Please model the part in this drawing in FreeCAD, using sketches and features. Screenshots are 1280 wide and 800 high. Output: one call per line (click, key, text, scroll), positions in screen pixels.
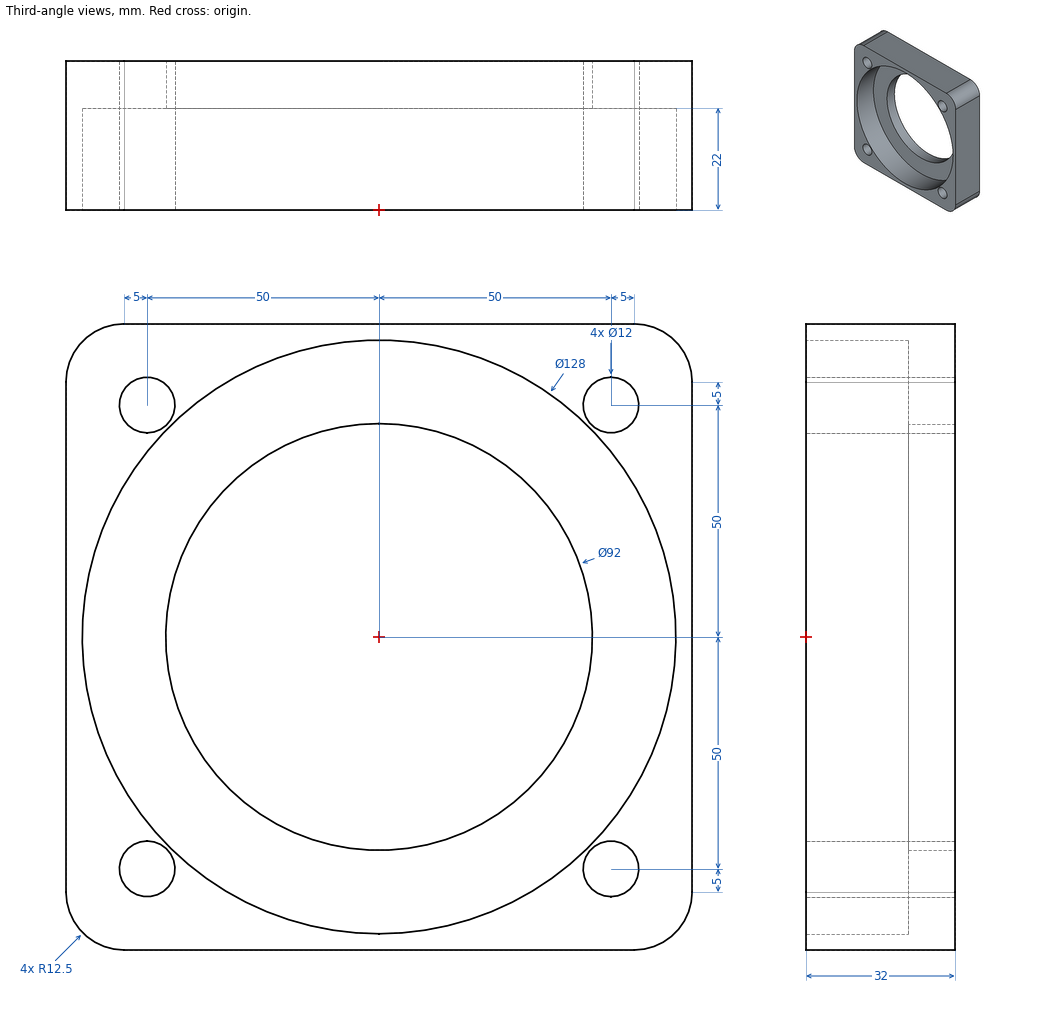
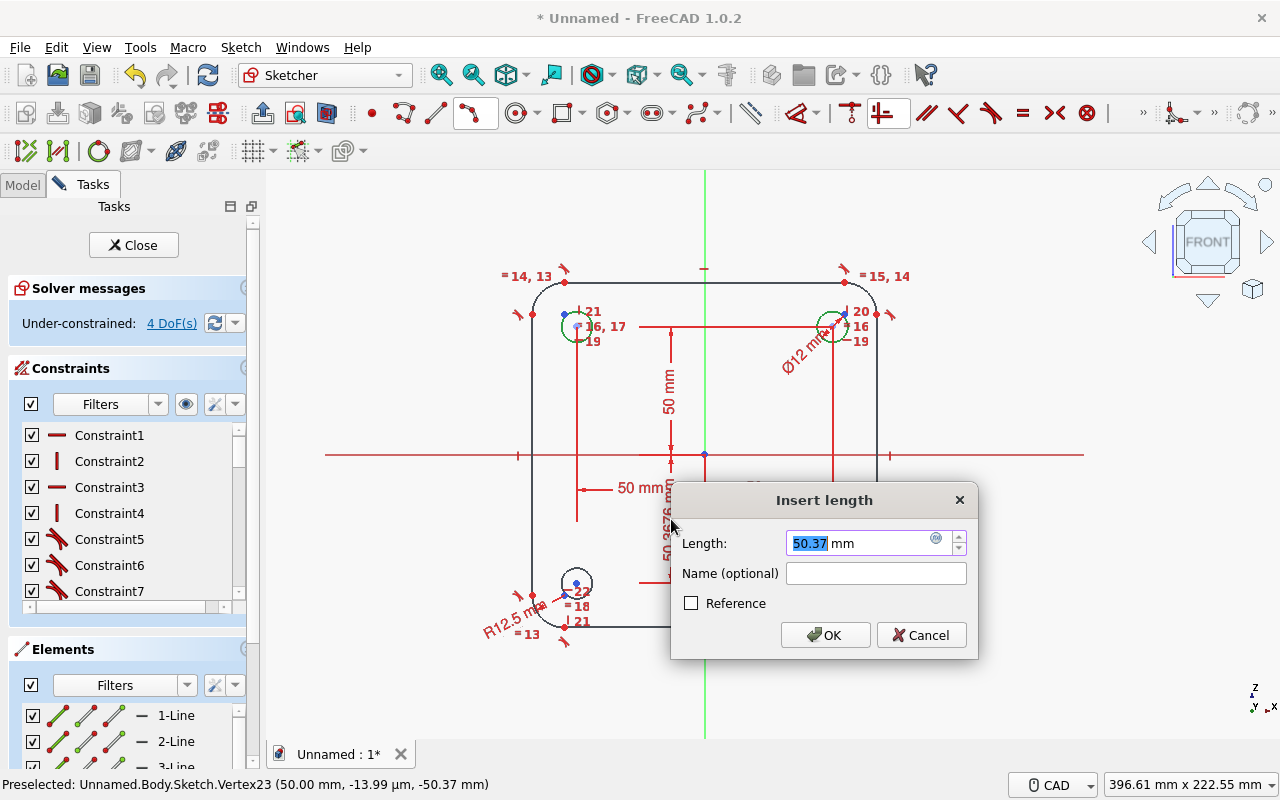
text(50)
key(Return)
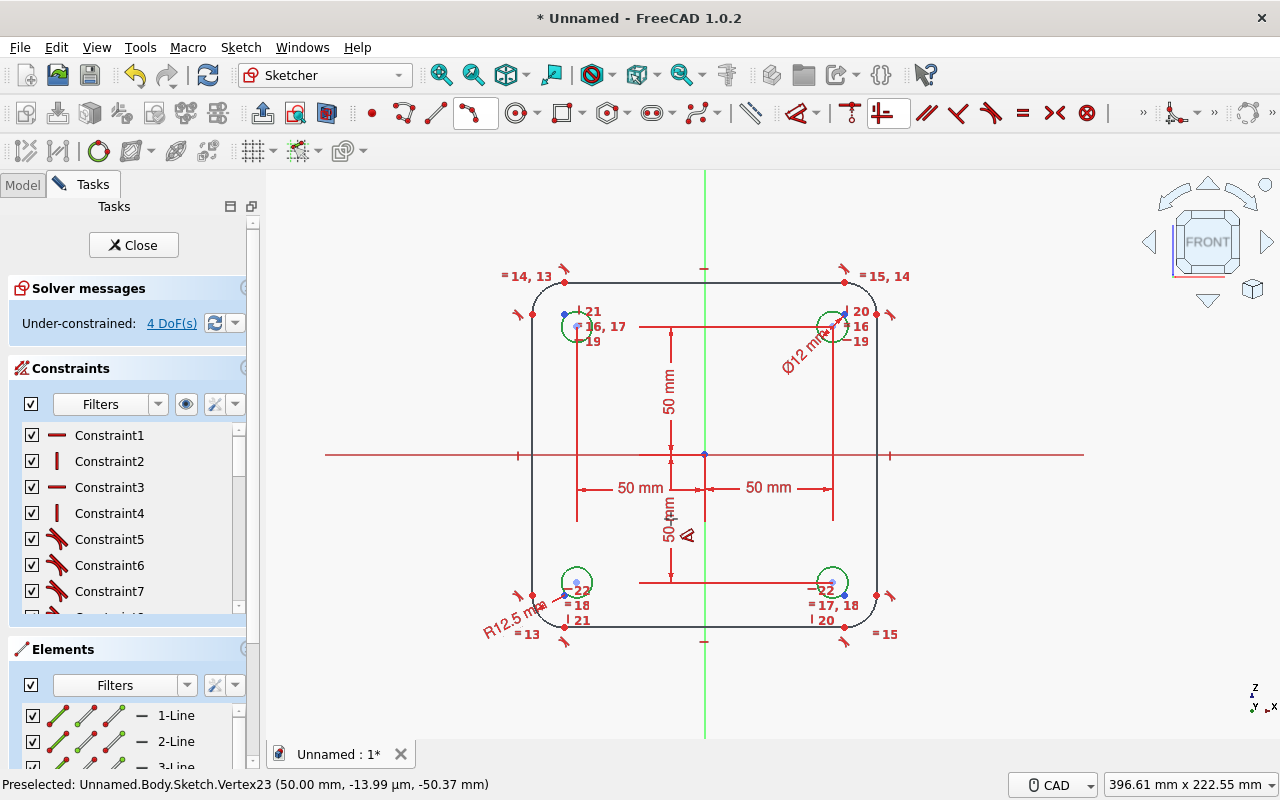
scroll(845, 283, up, 6)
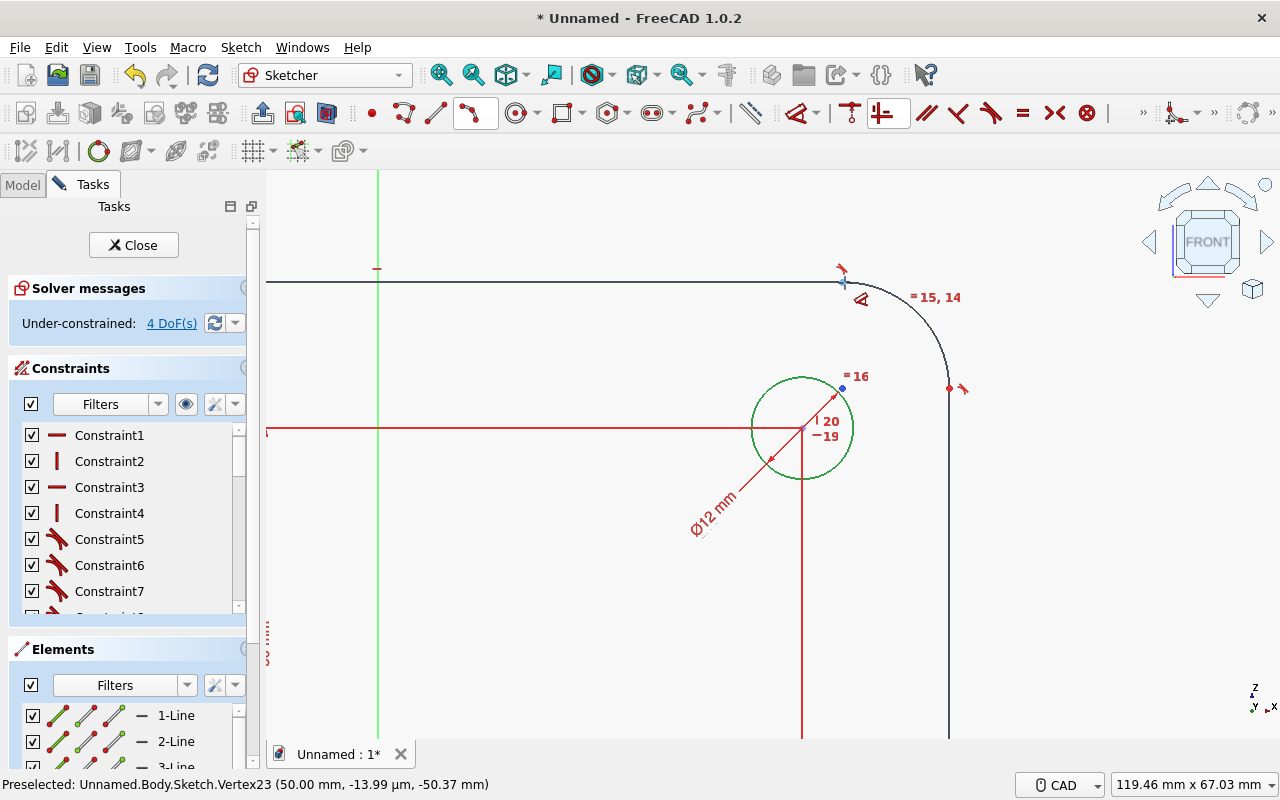
click(843, 282)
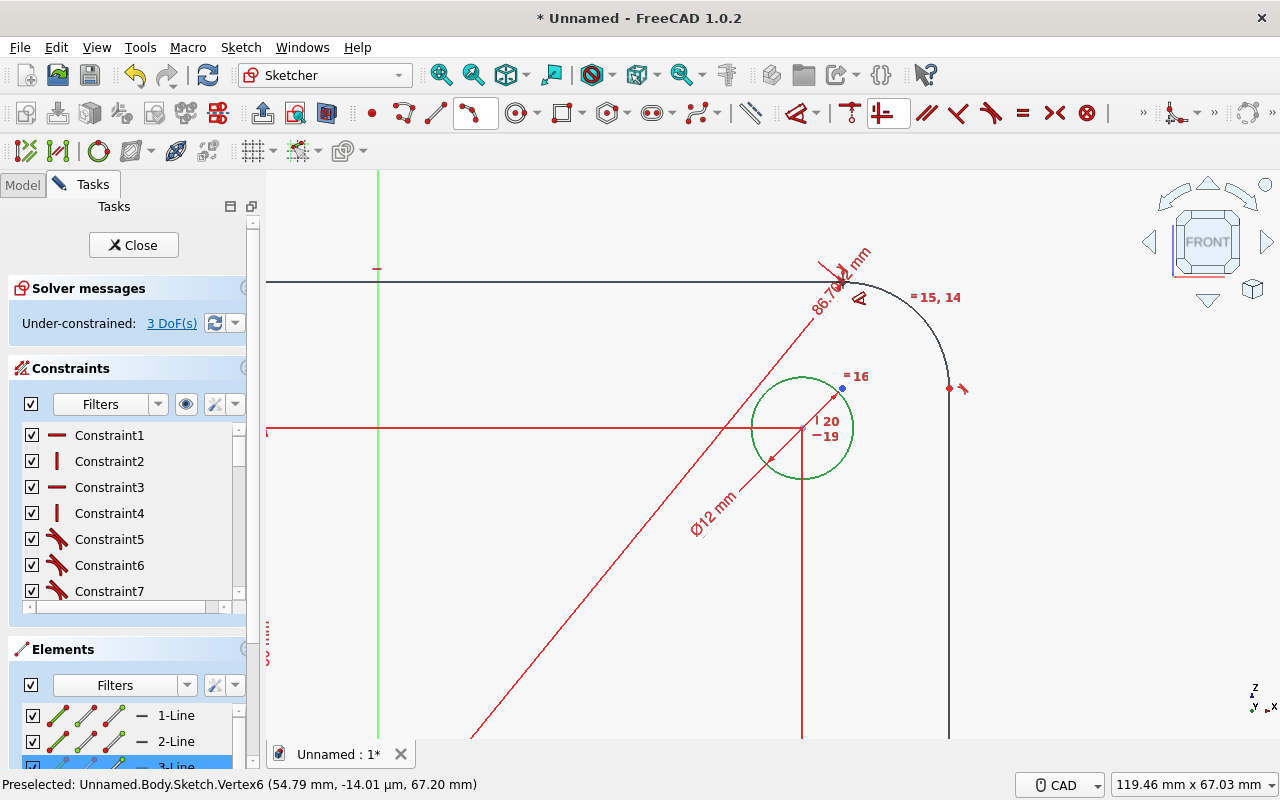
click(802, 428)
click(823, 248)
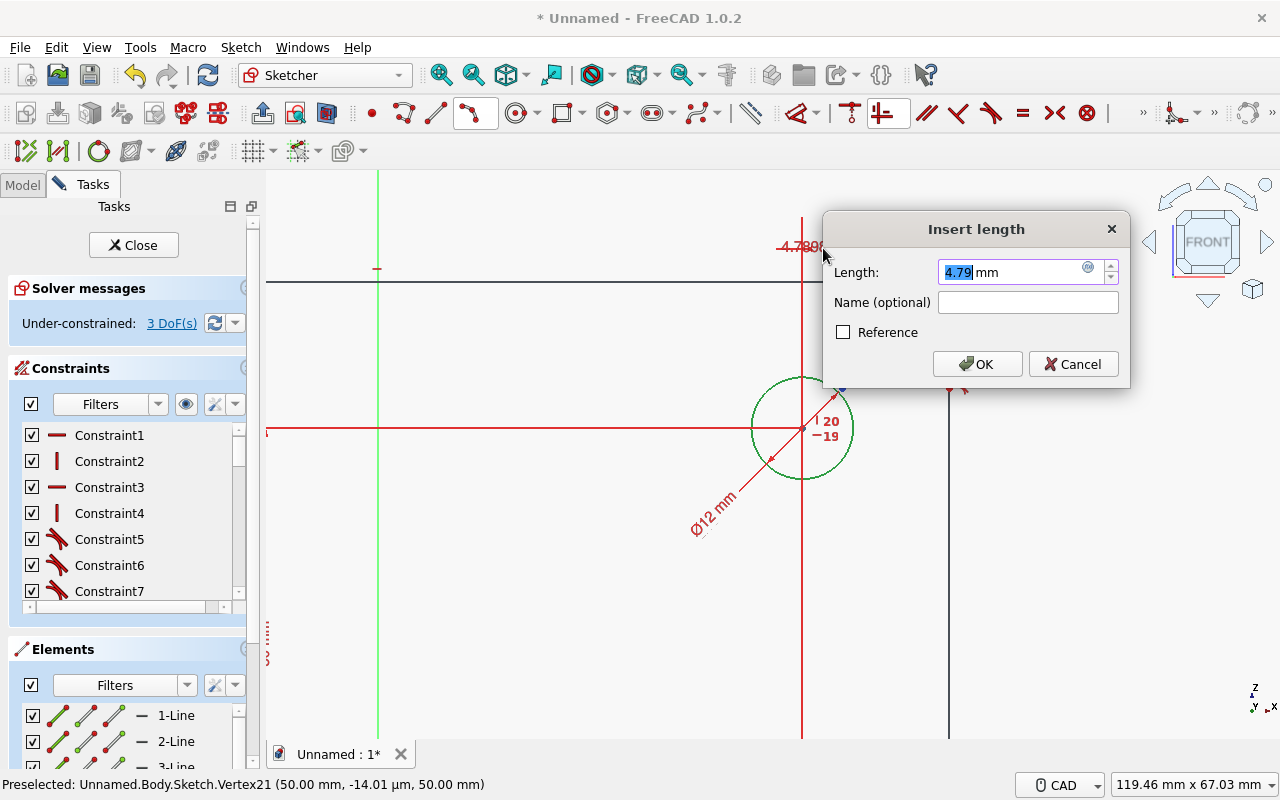
text(5)
key(Return)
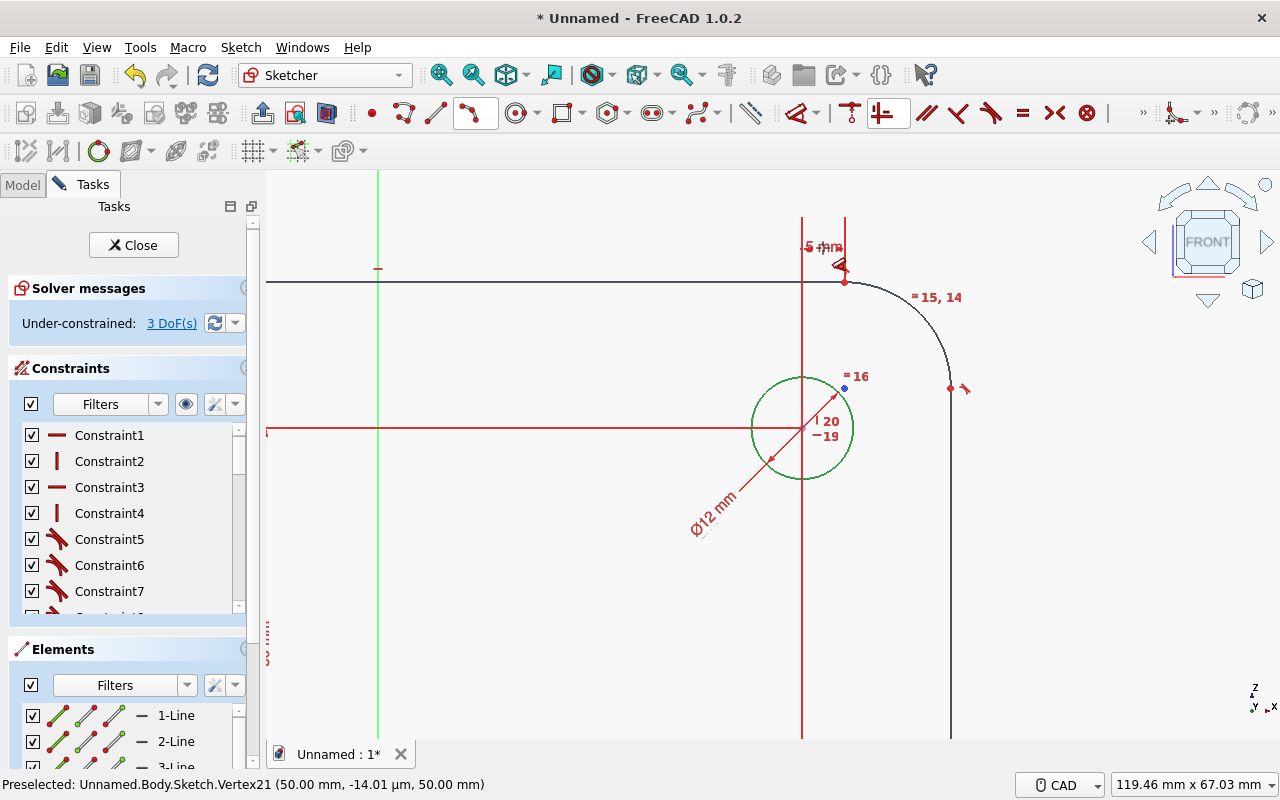
click(951, 388)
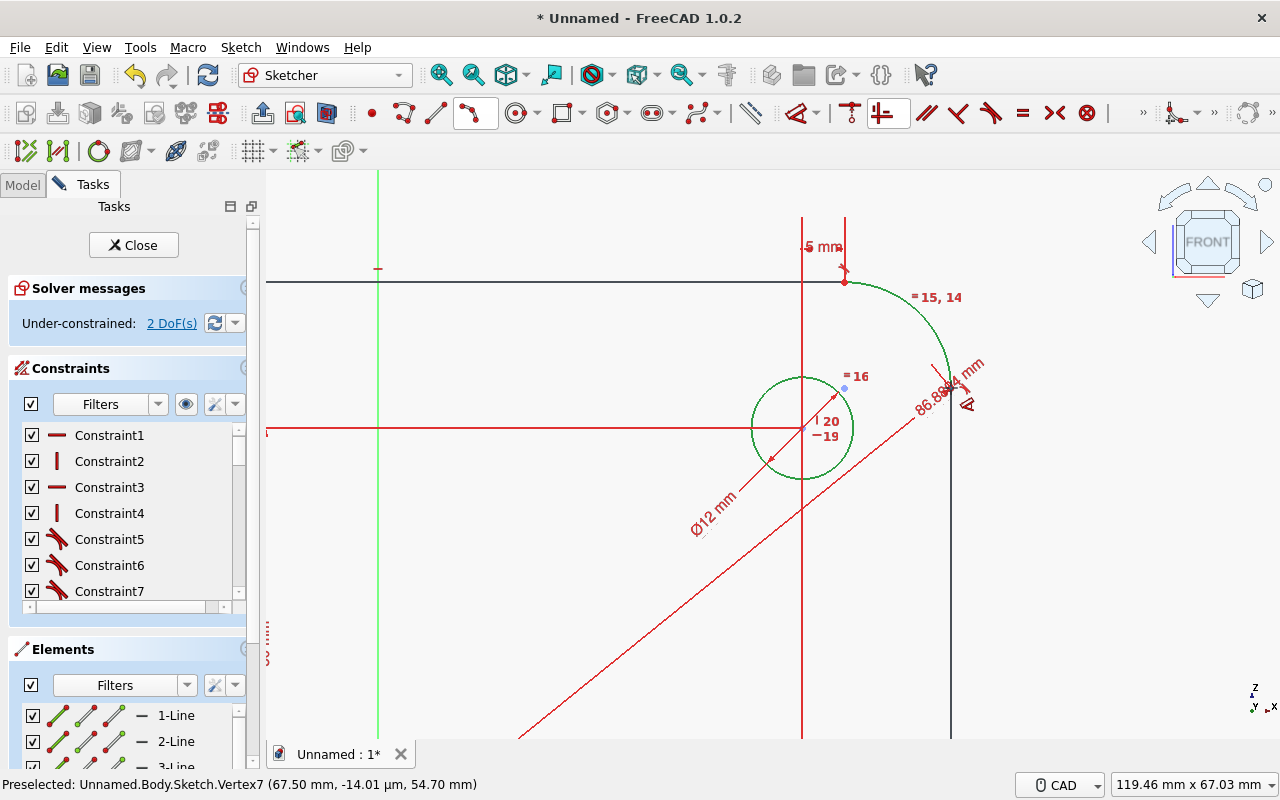
click(802, 428)
click(985, 408)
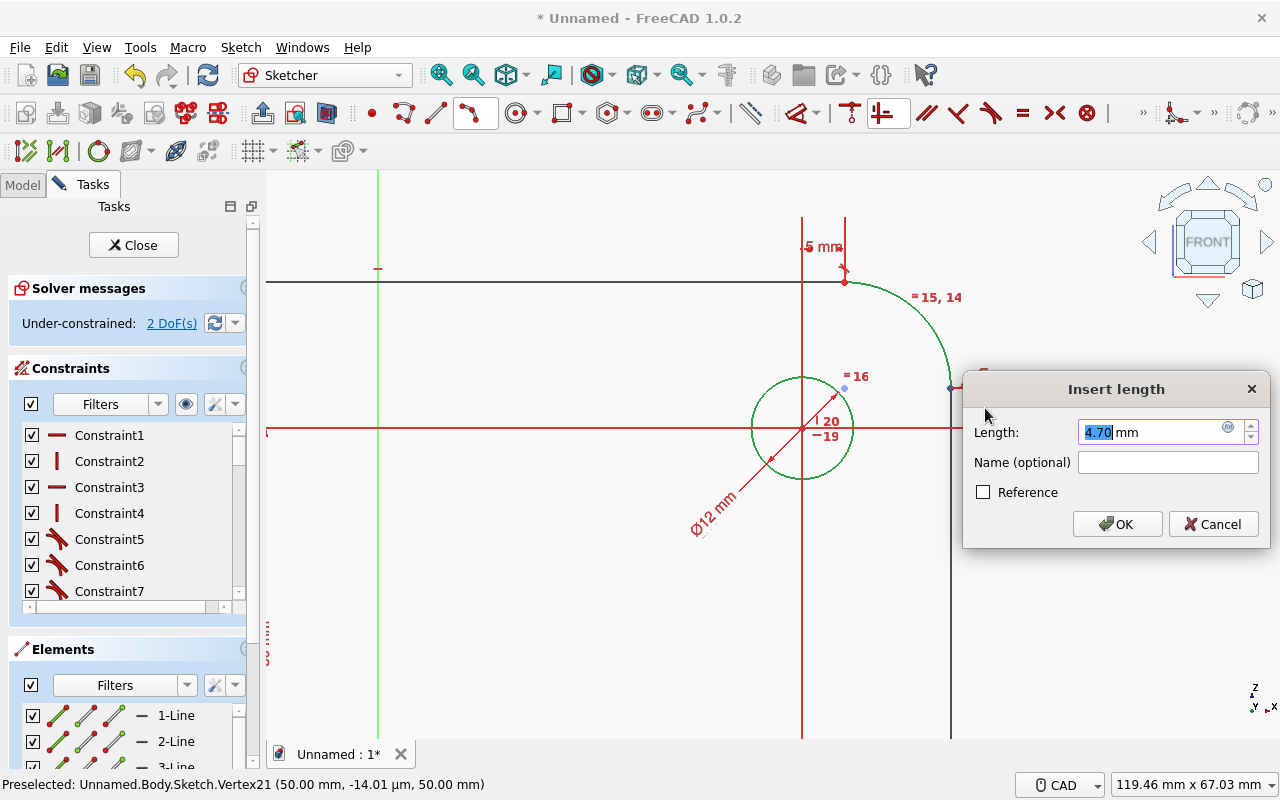
text(5)
key(Return)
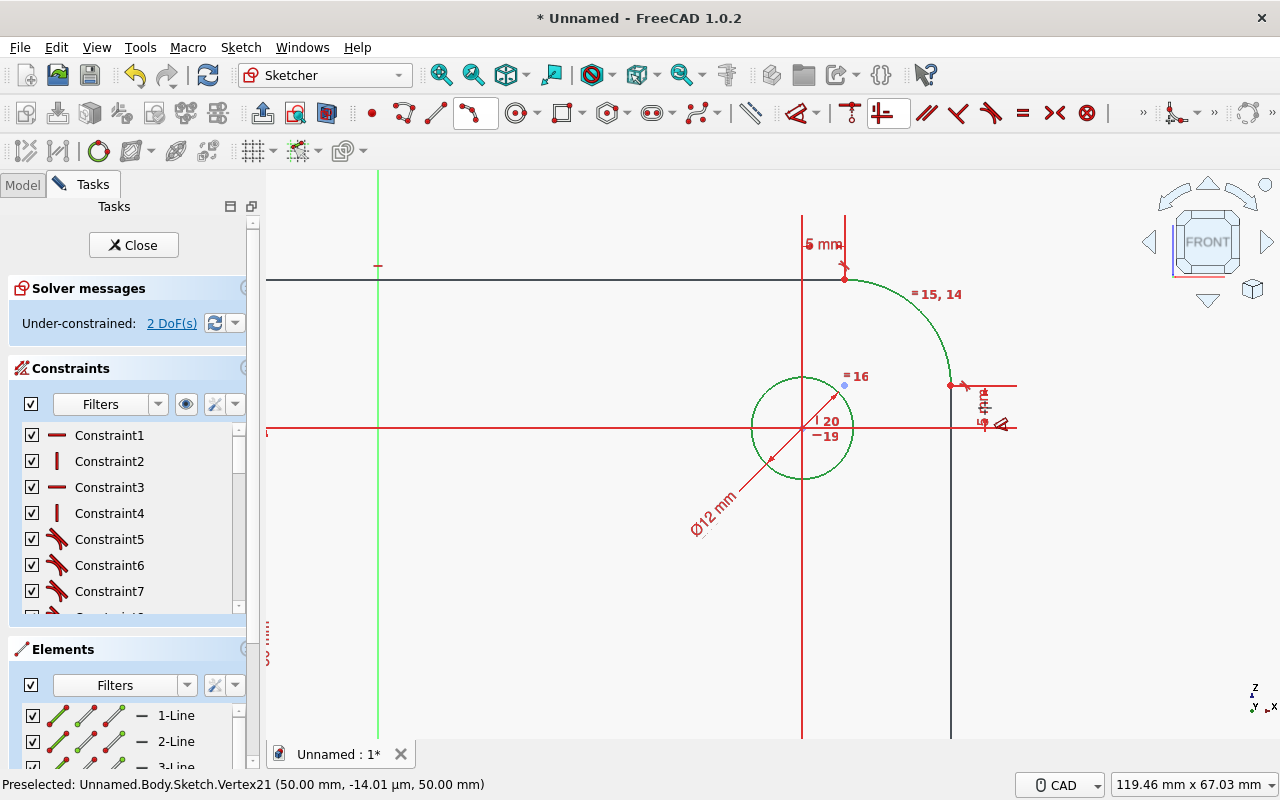
scroll(845, 283, down, 6)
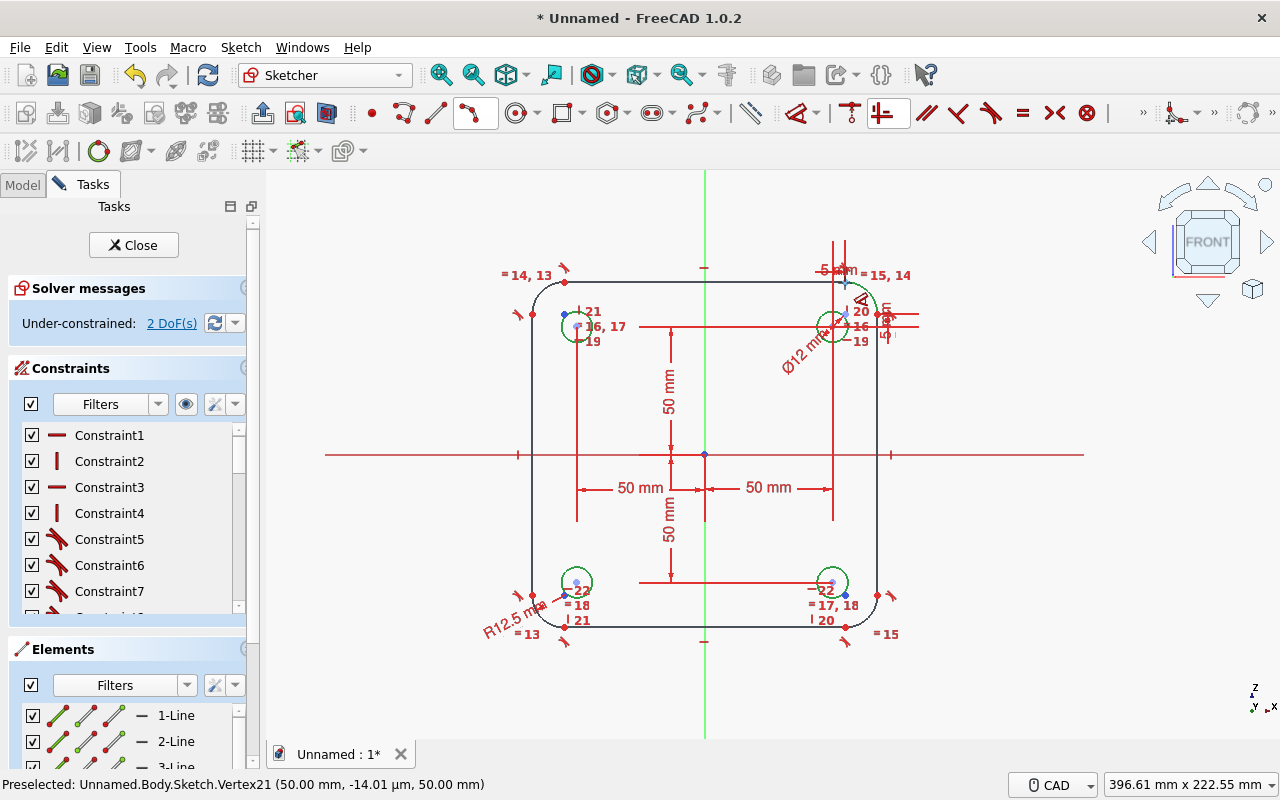
scroll(564, 282, up, 6)